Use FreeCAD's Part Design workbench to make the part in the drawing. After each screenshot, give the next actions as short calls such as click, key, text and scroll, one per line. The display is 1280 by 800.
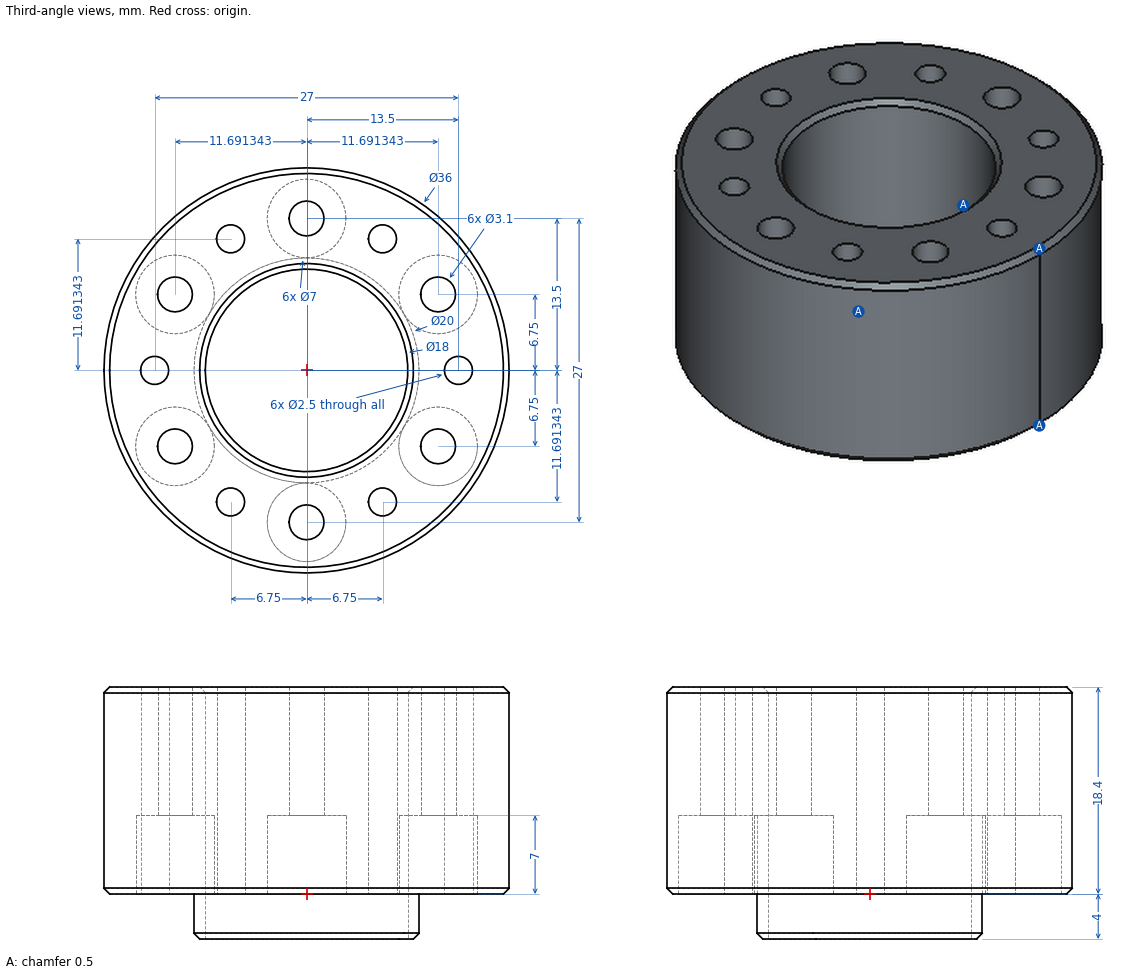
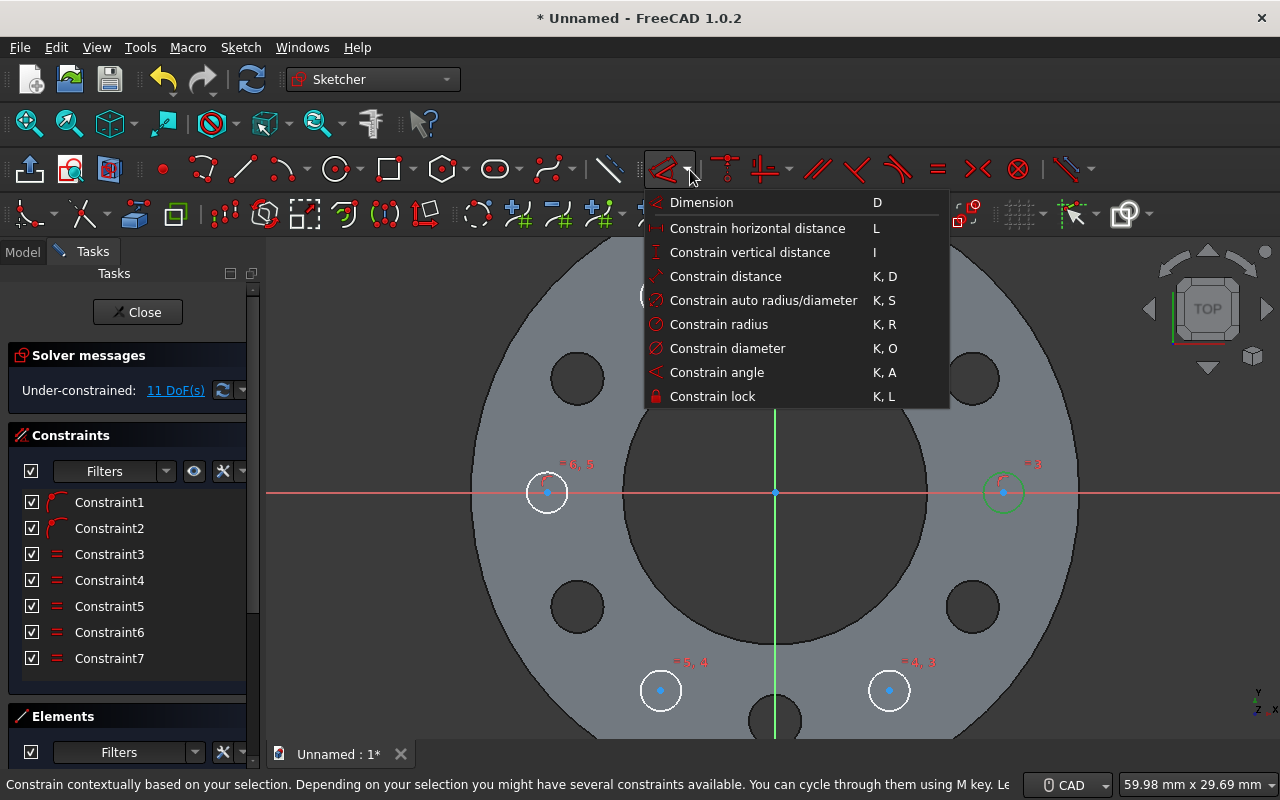
click(797, 348)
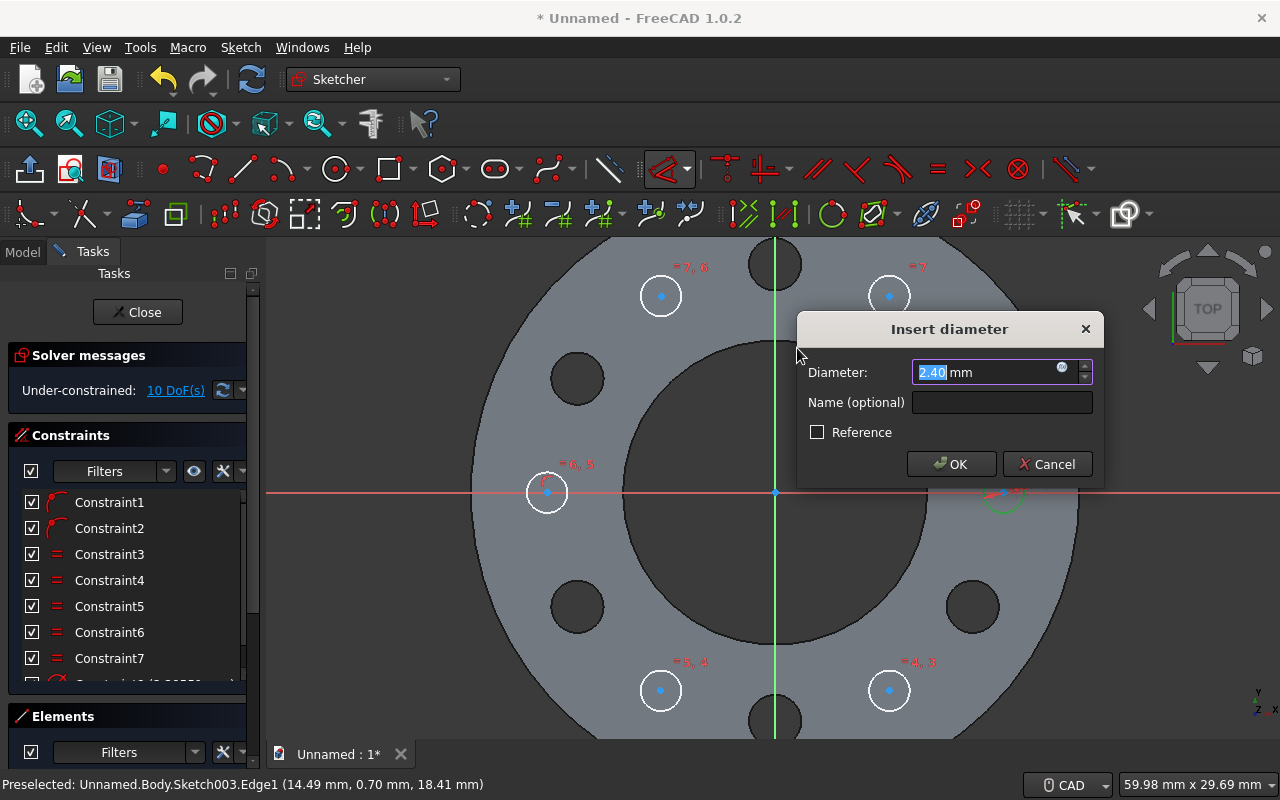
text(2.5)
key(Return)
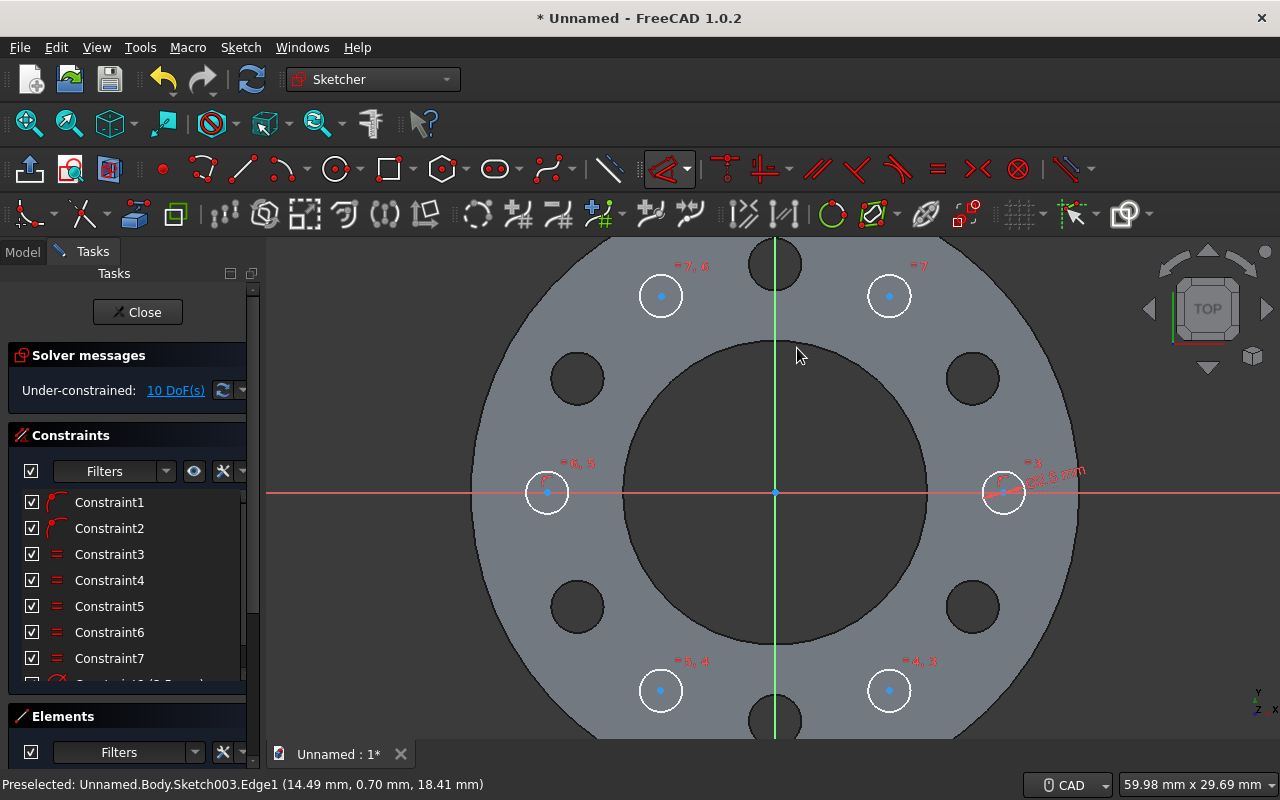
click(1004, 493)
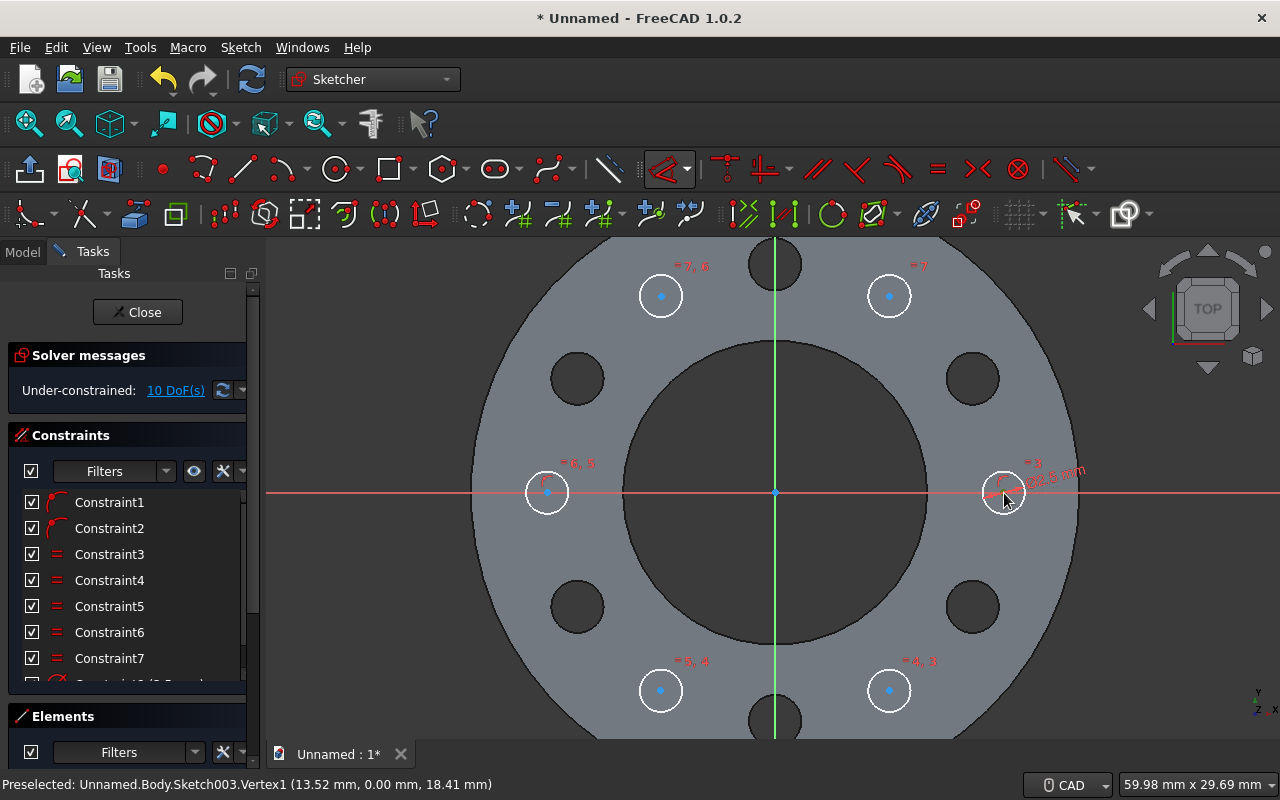
click(547, 493)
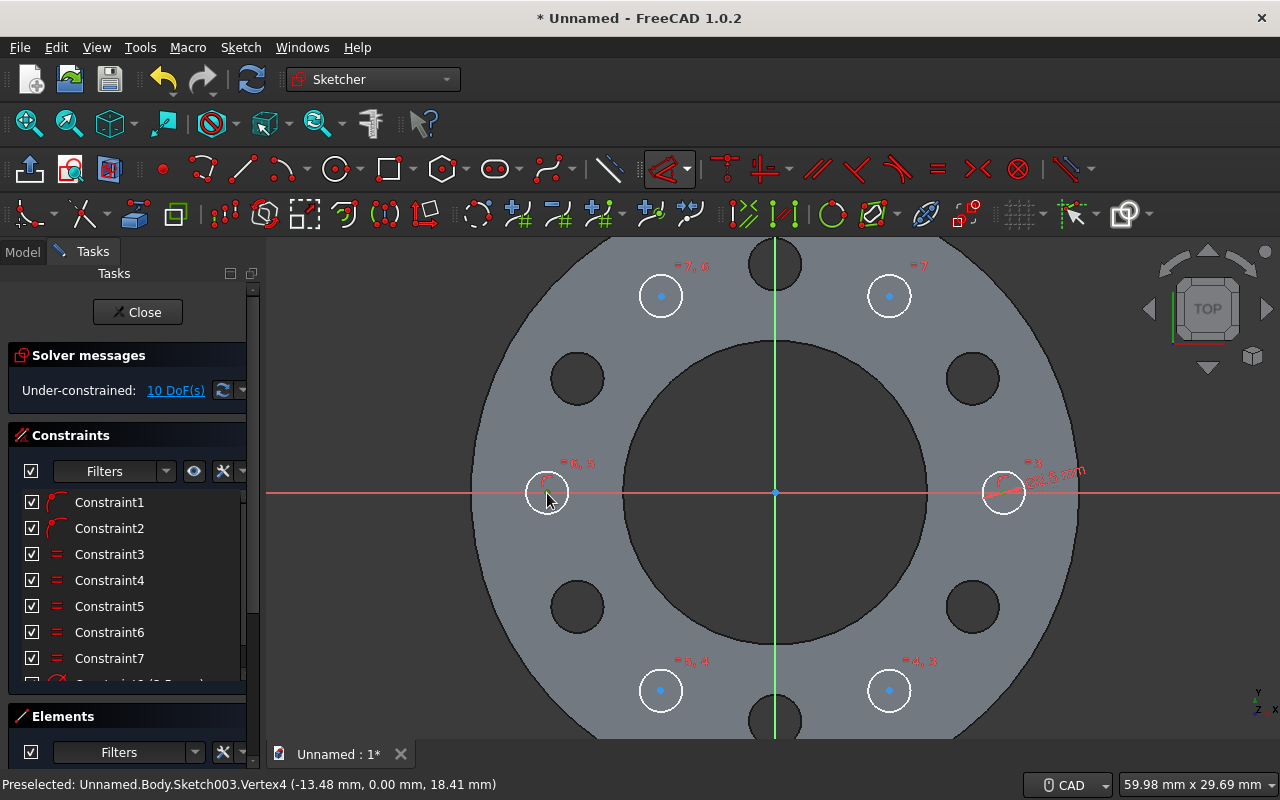
click(690, 170)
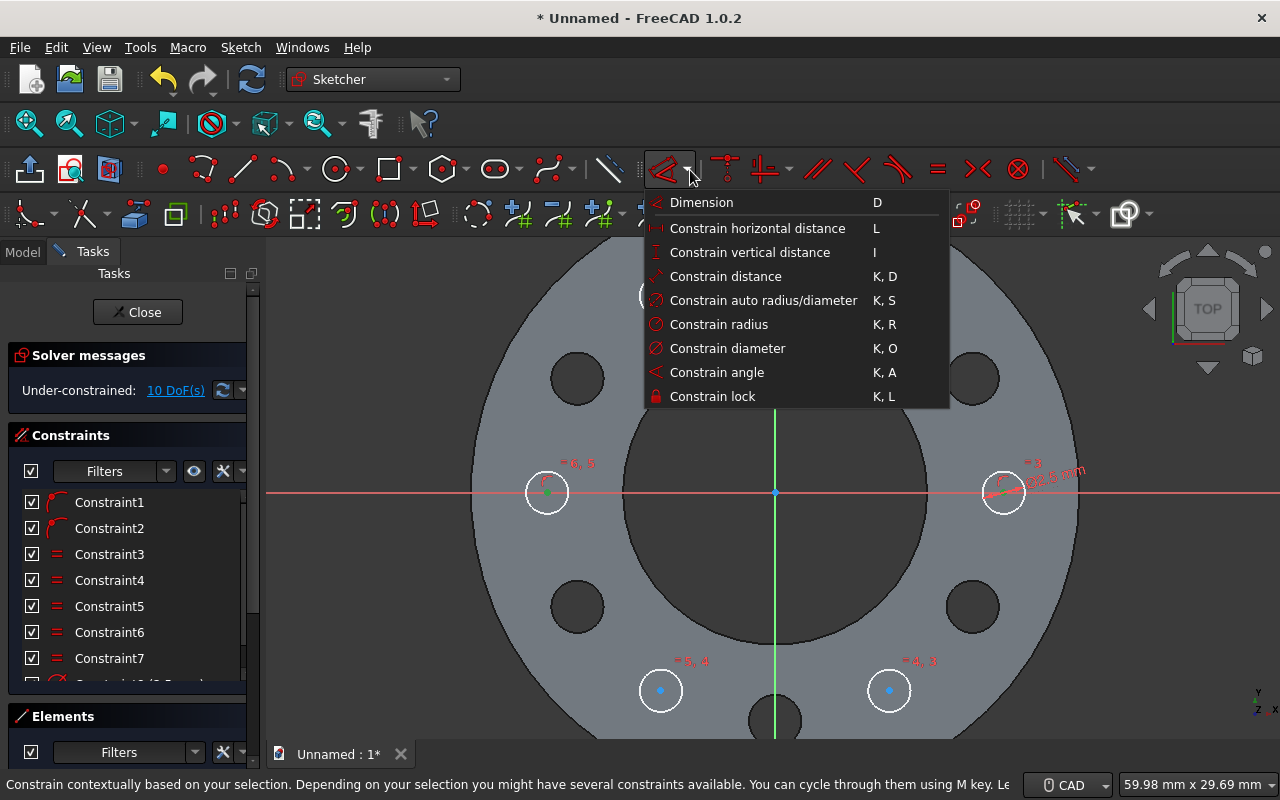
click(797, 228)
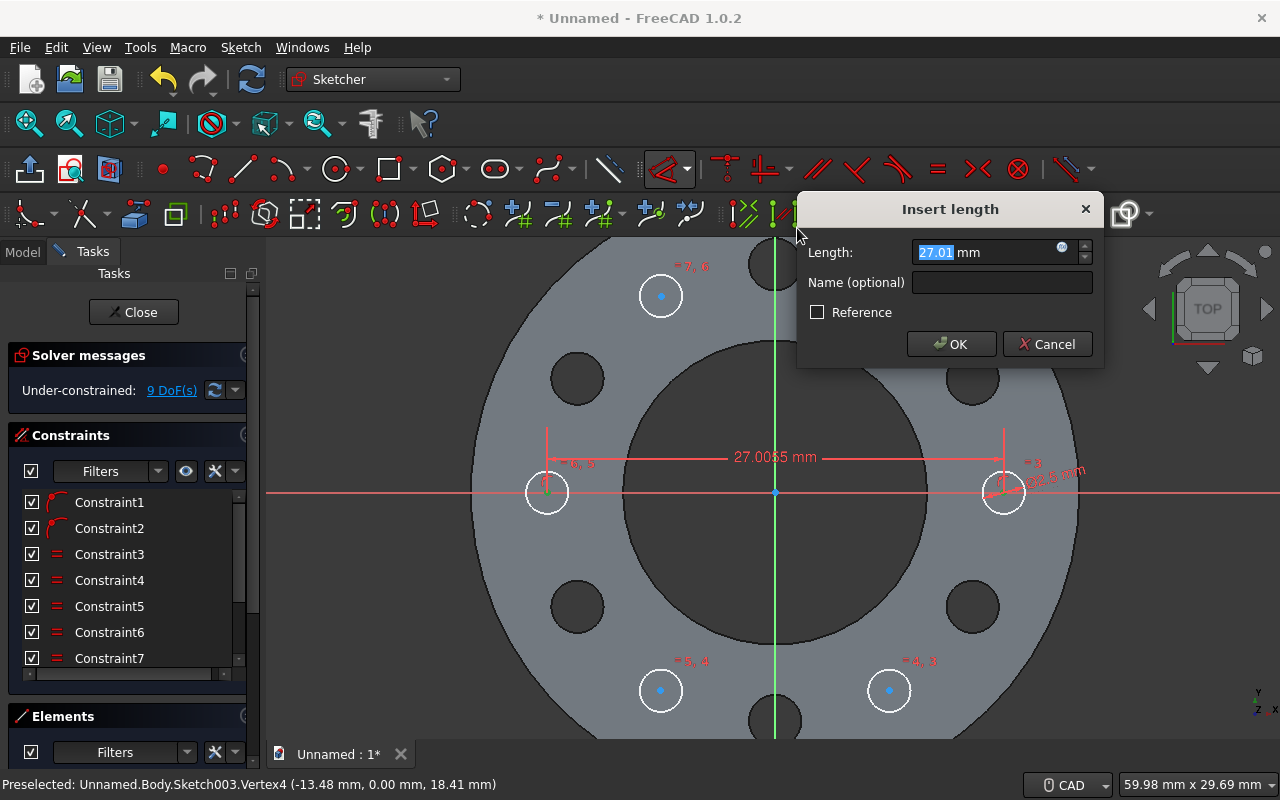
text(27)
key(Return)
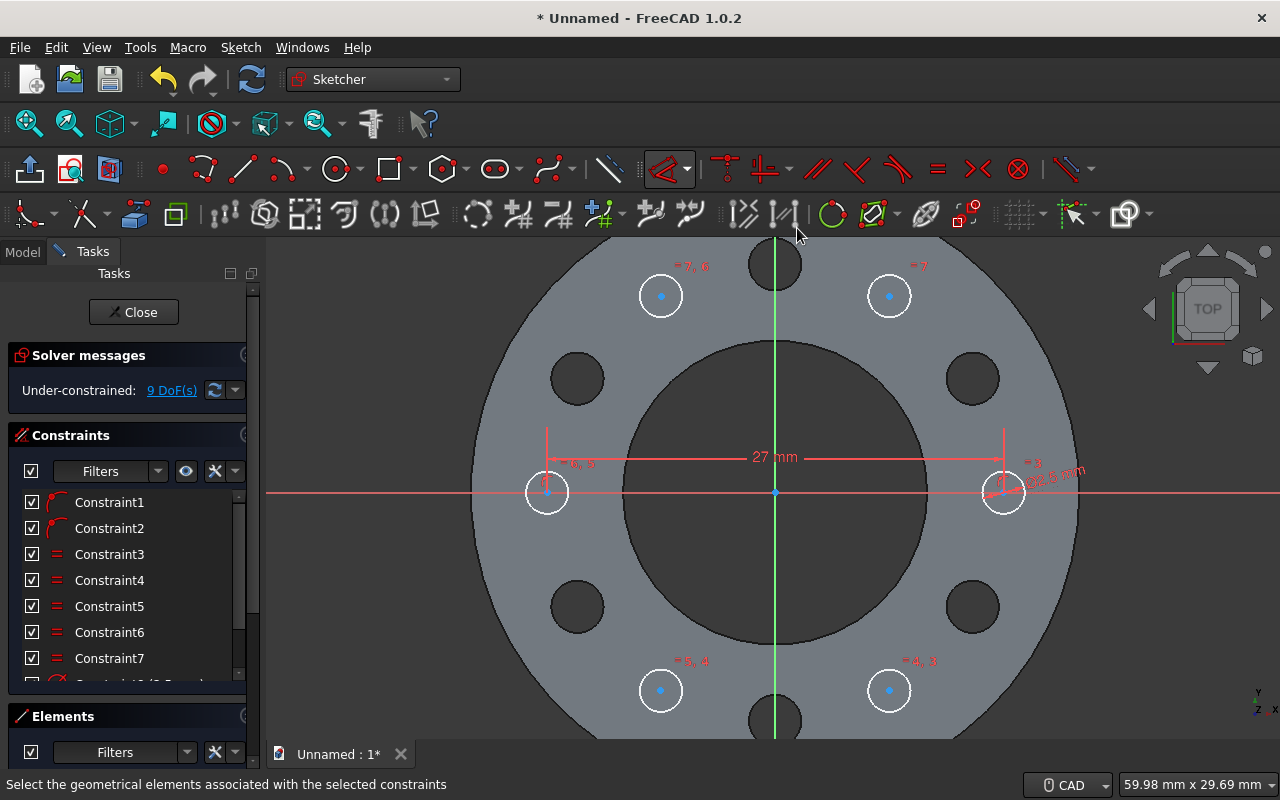
click(1004, 493)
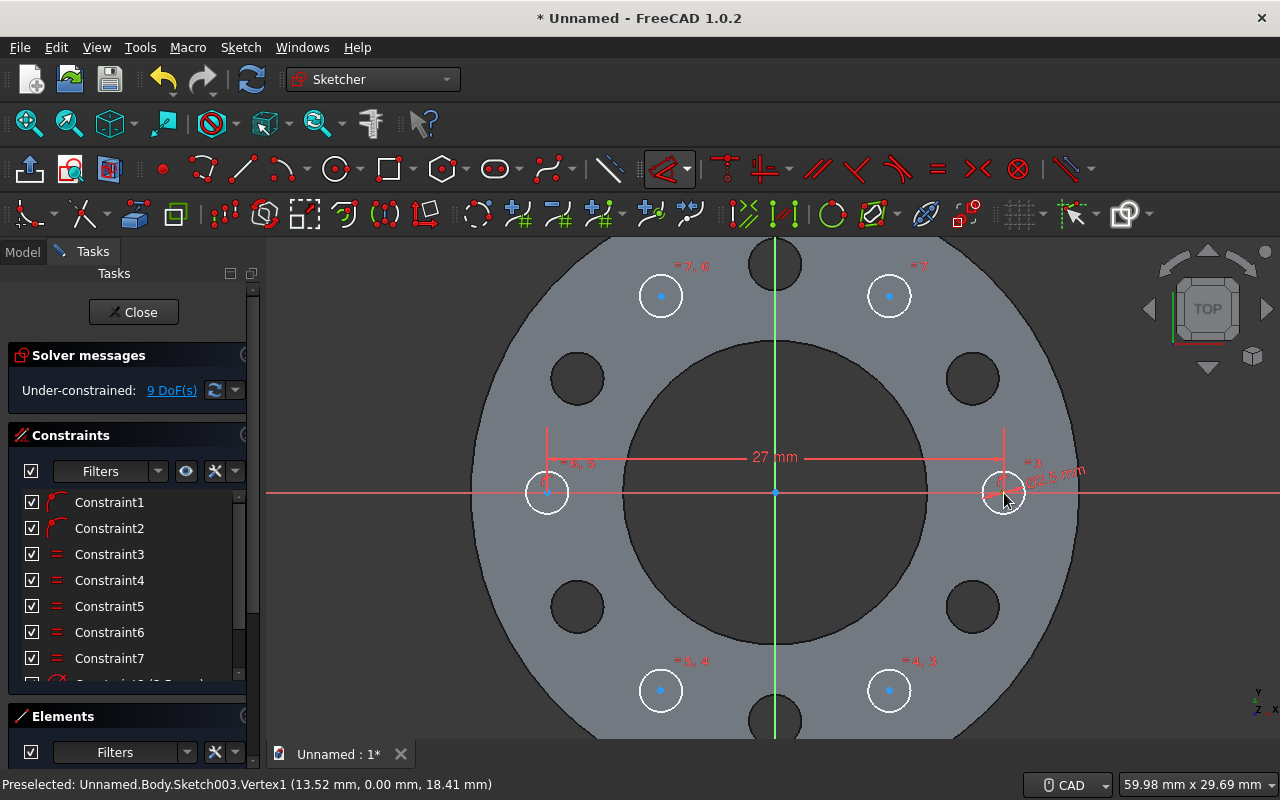
click(690, 170)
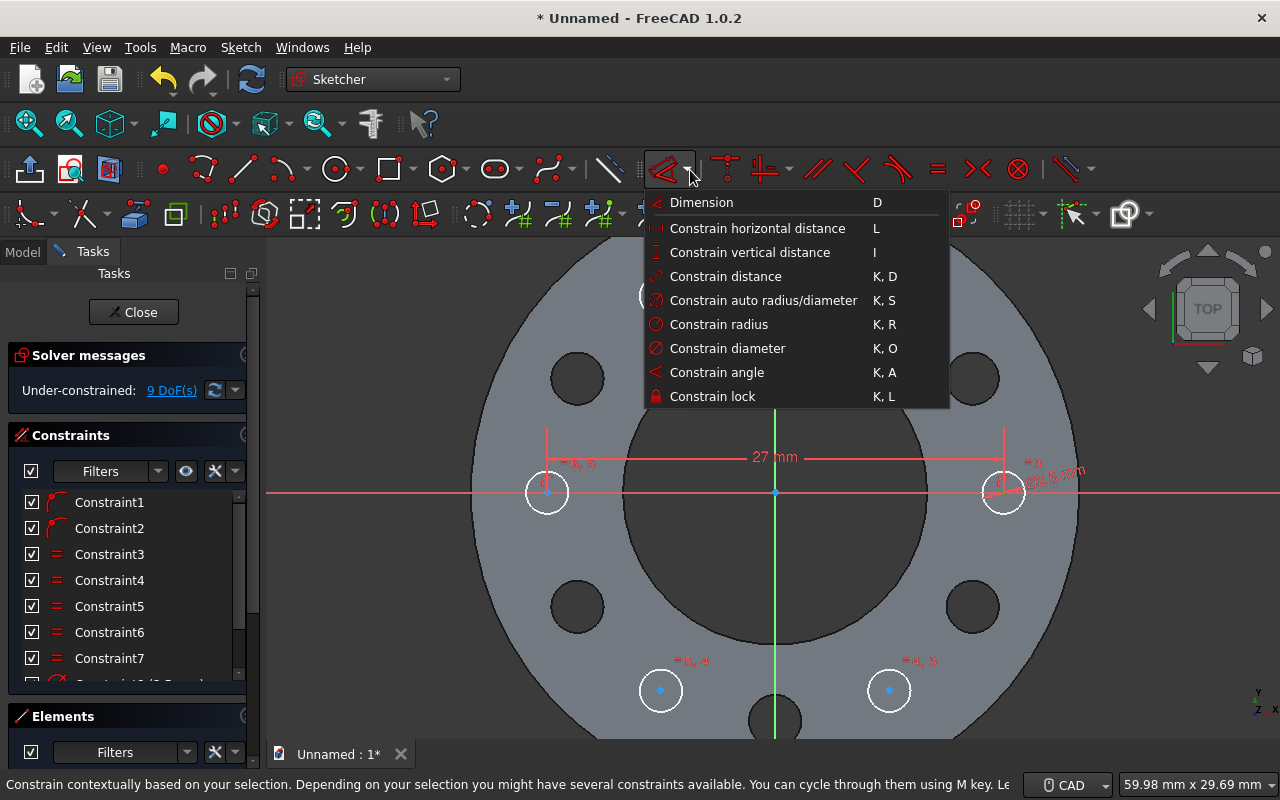
click(797, 228)